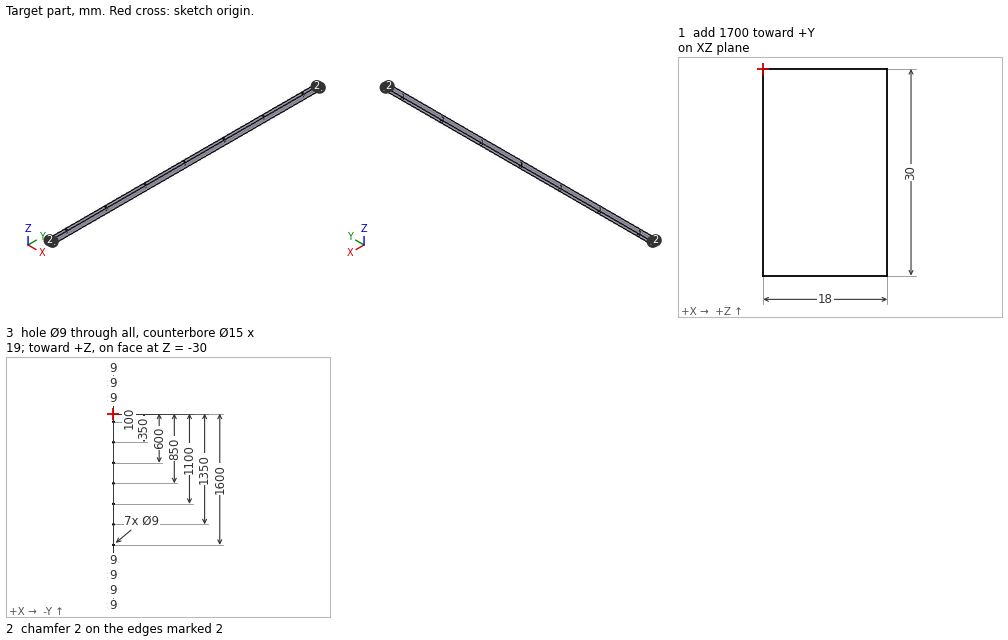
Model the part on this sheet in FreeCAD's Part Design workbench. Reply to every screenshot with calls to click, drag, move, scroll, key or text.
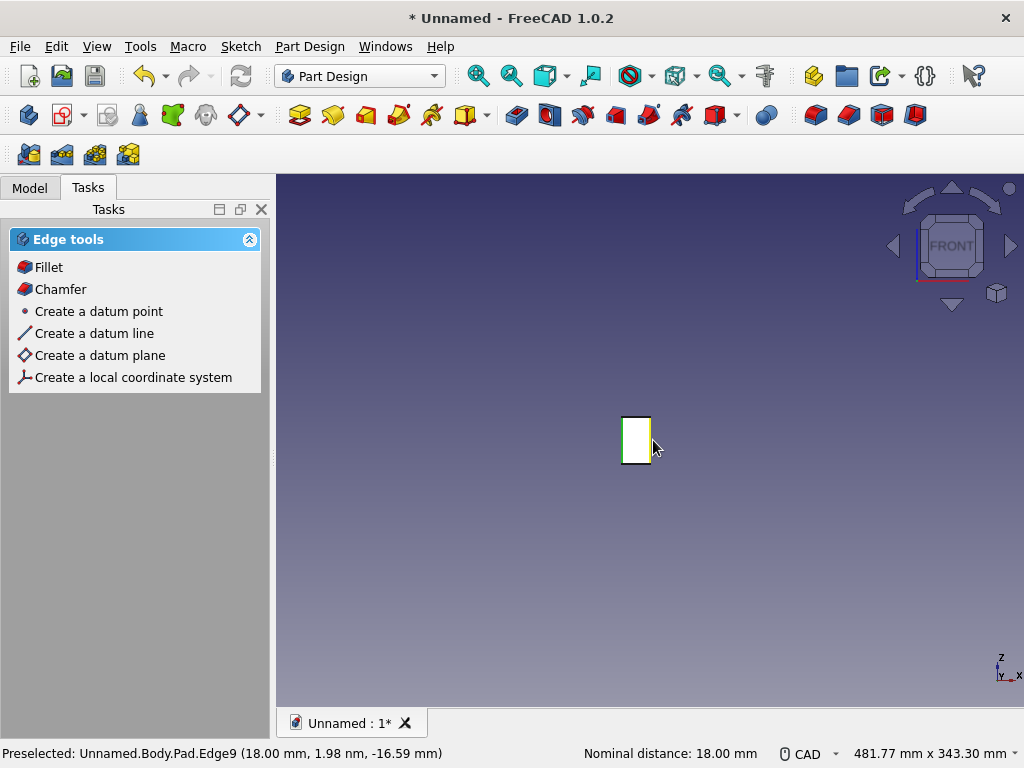
key(v)
key(f)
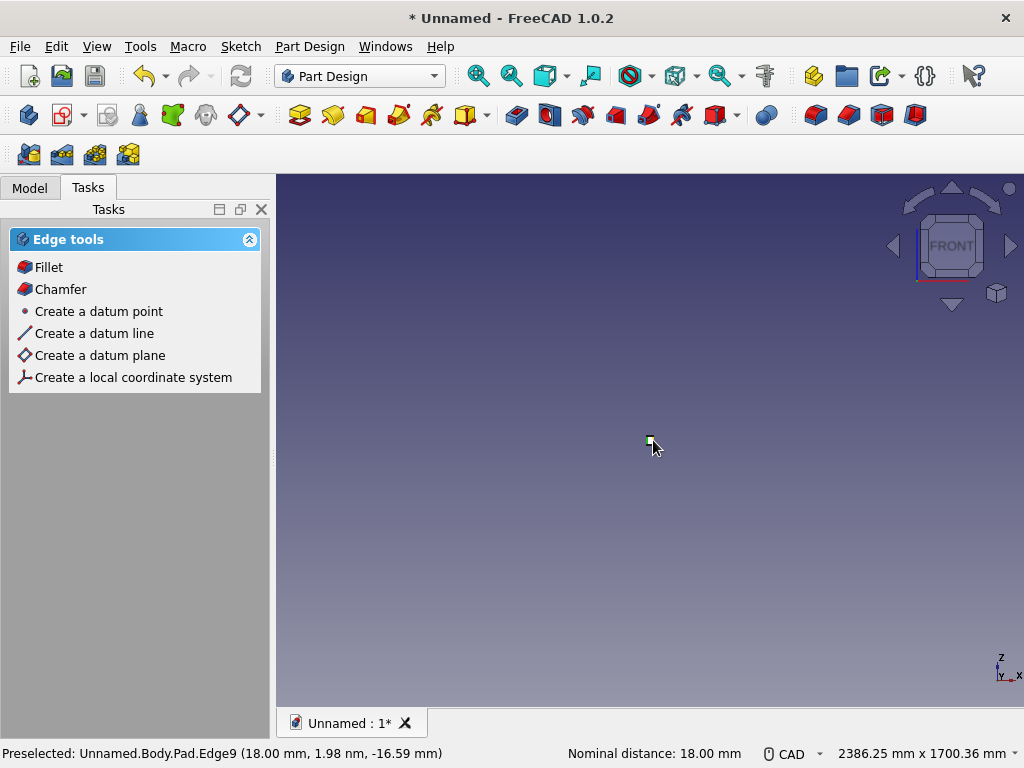
key(3)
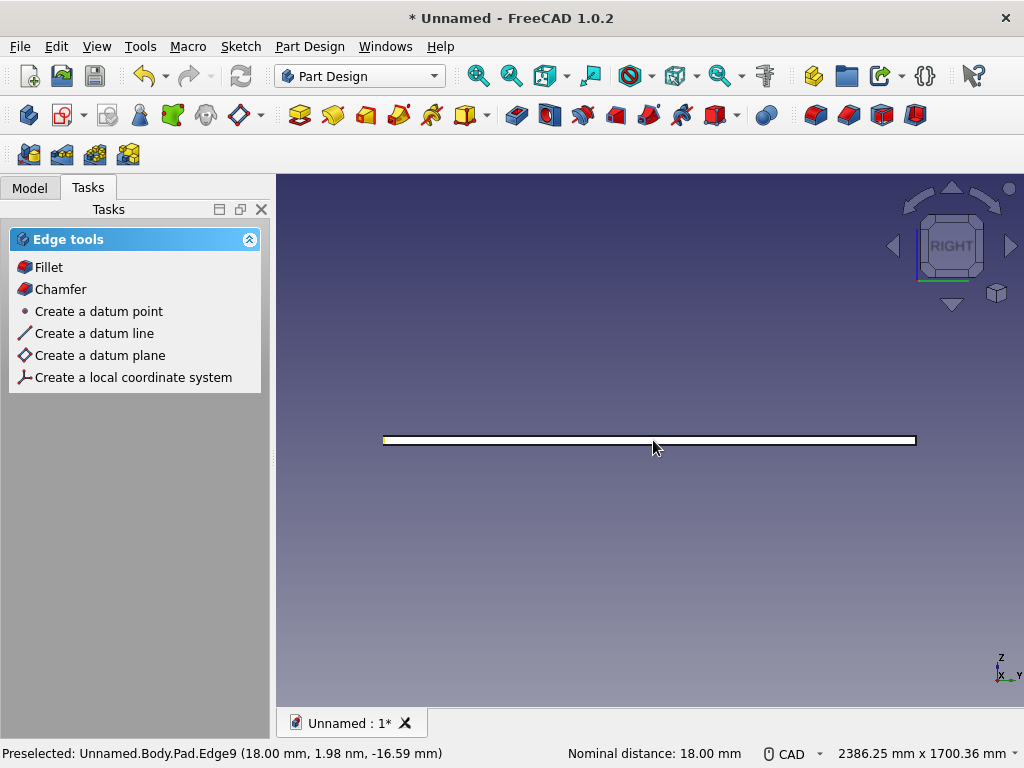
key(5)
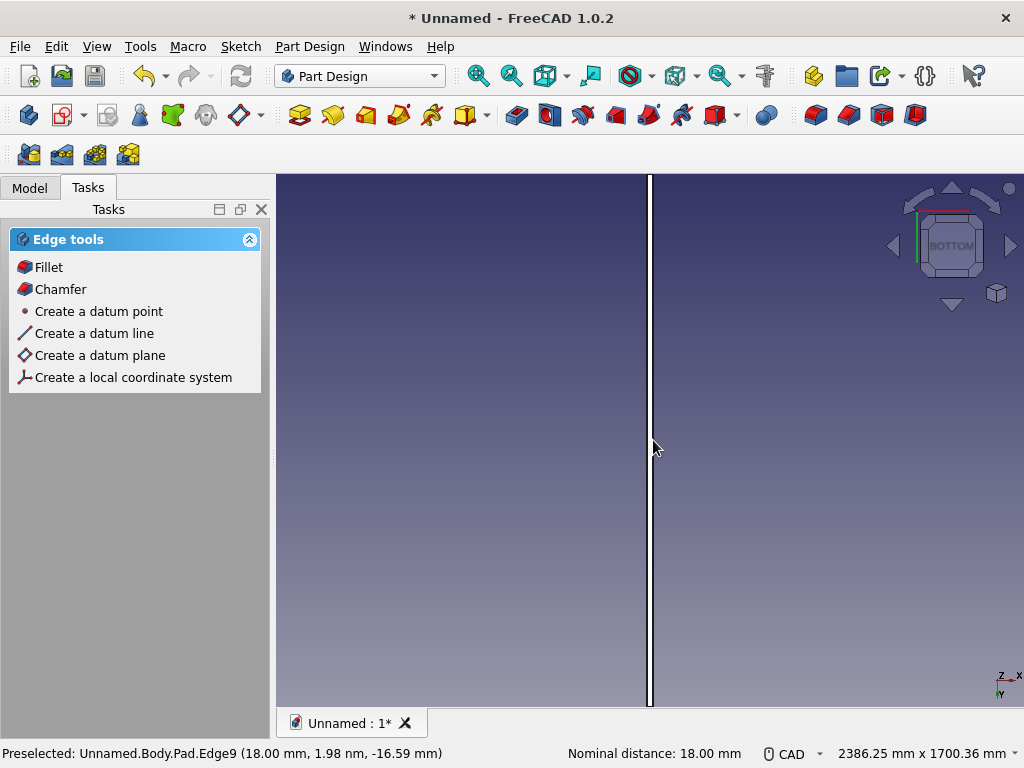
key(v)
key(f)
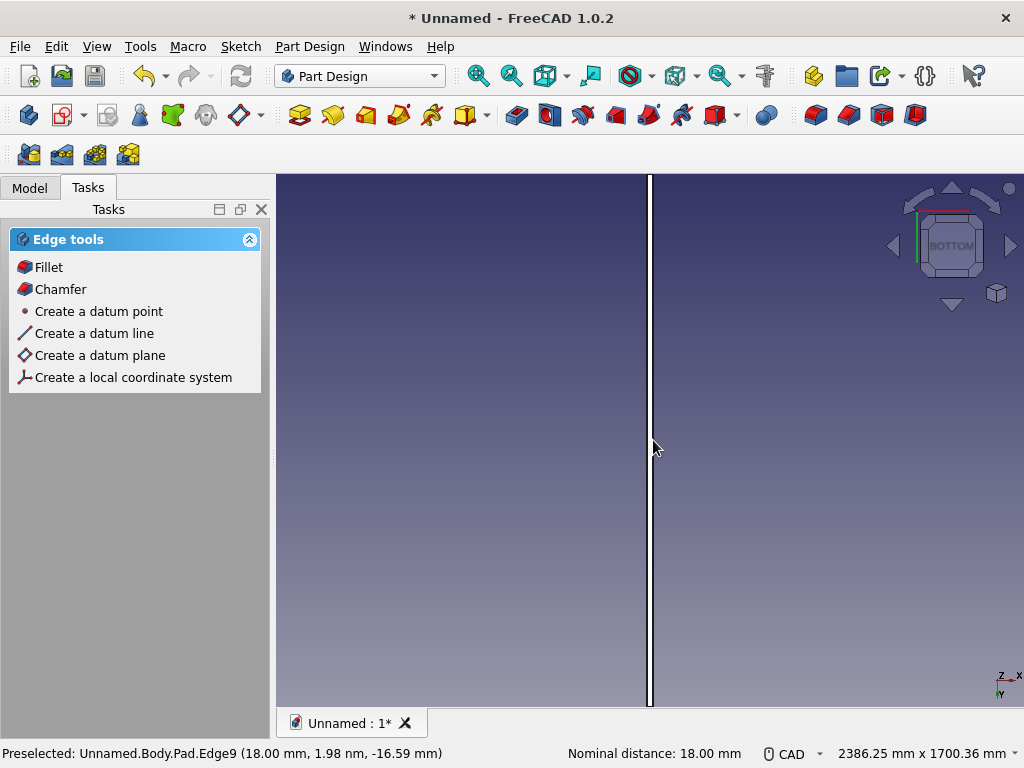
key(4)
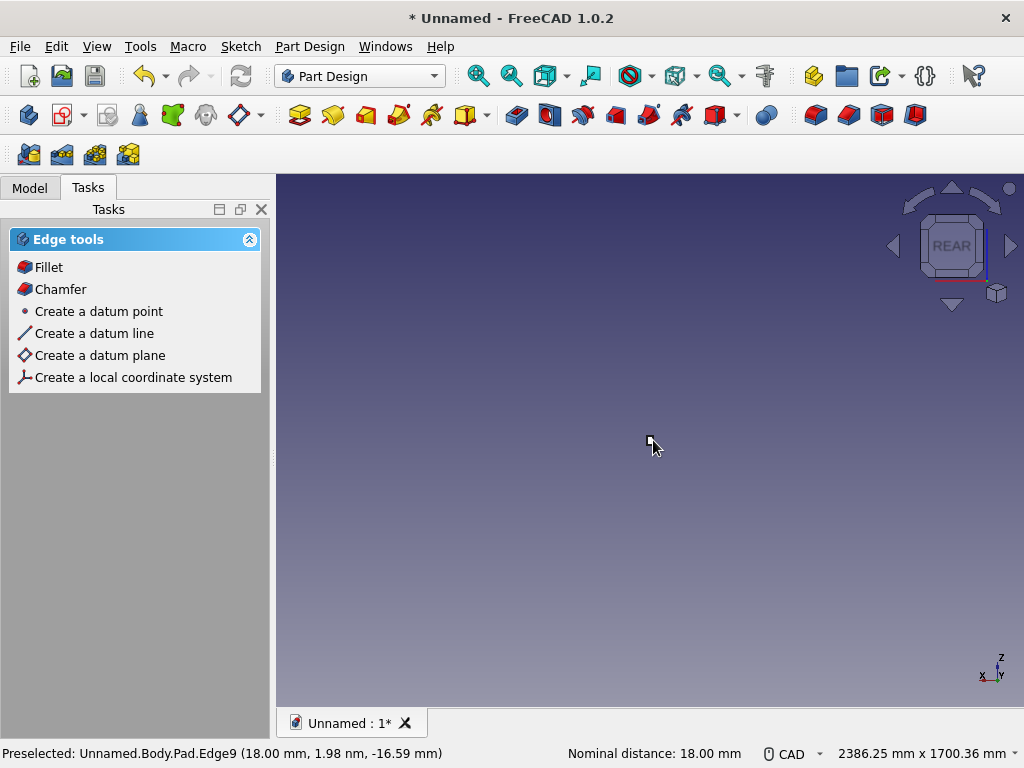
key(v)
key(f)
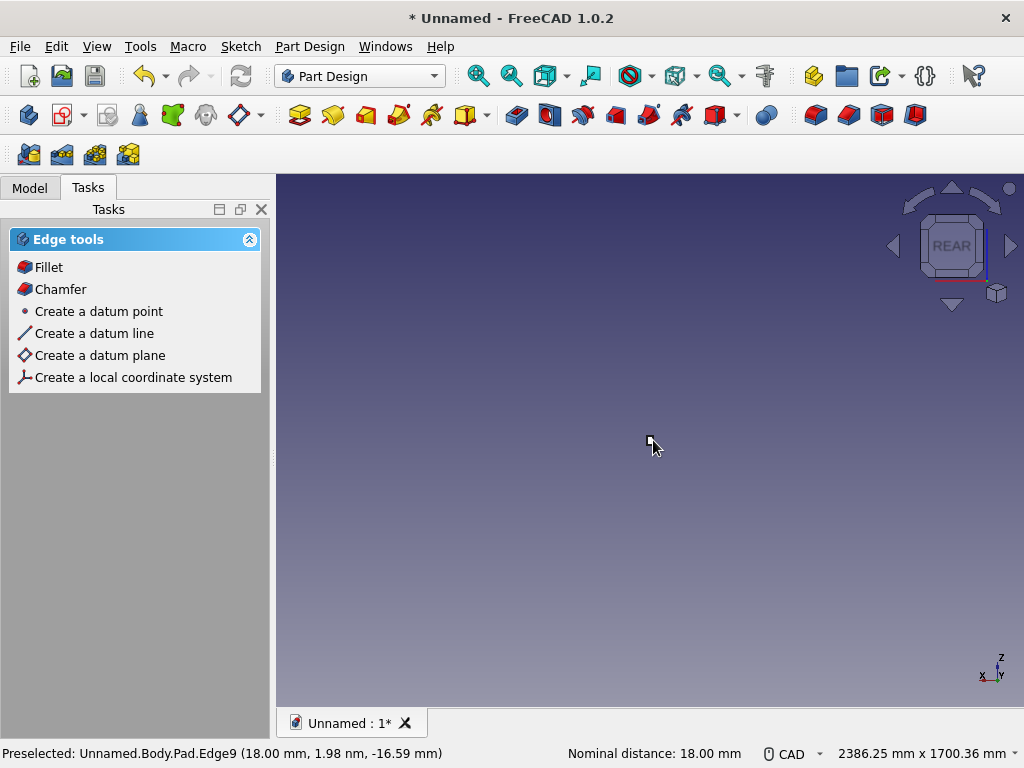
click(653, 438, ctrl)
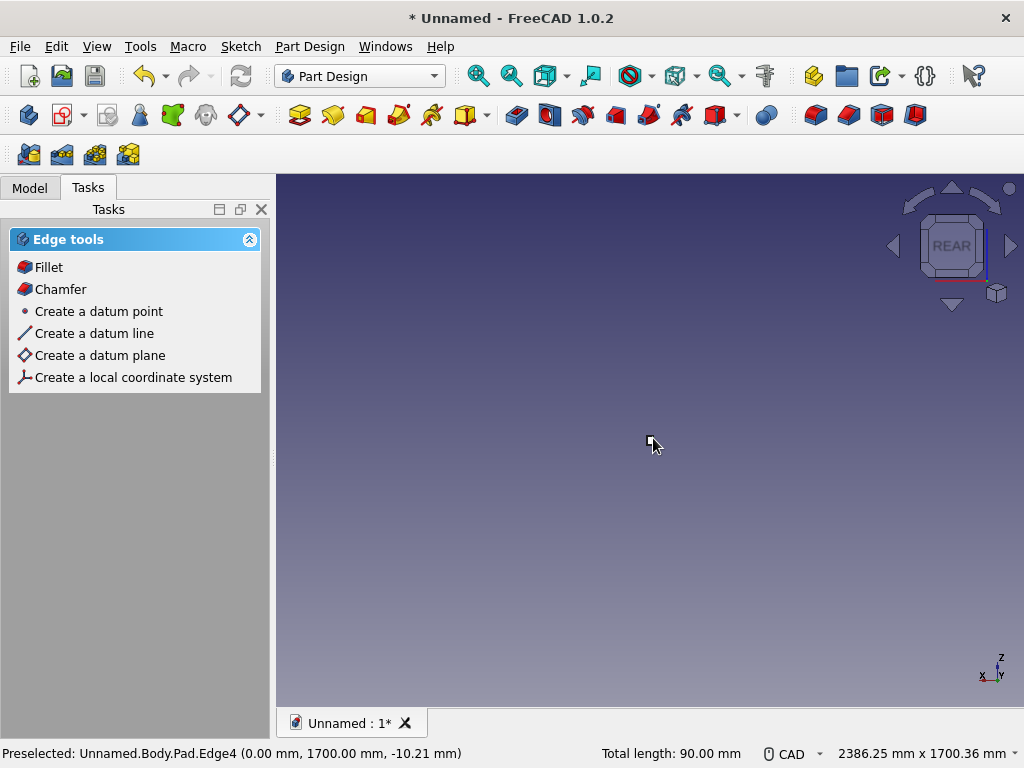
scroll(647, 440, up, 8)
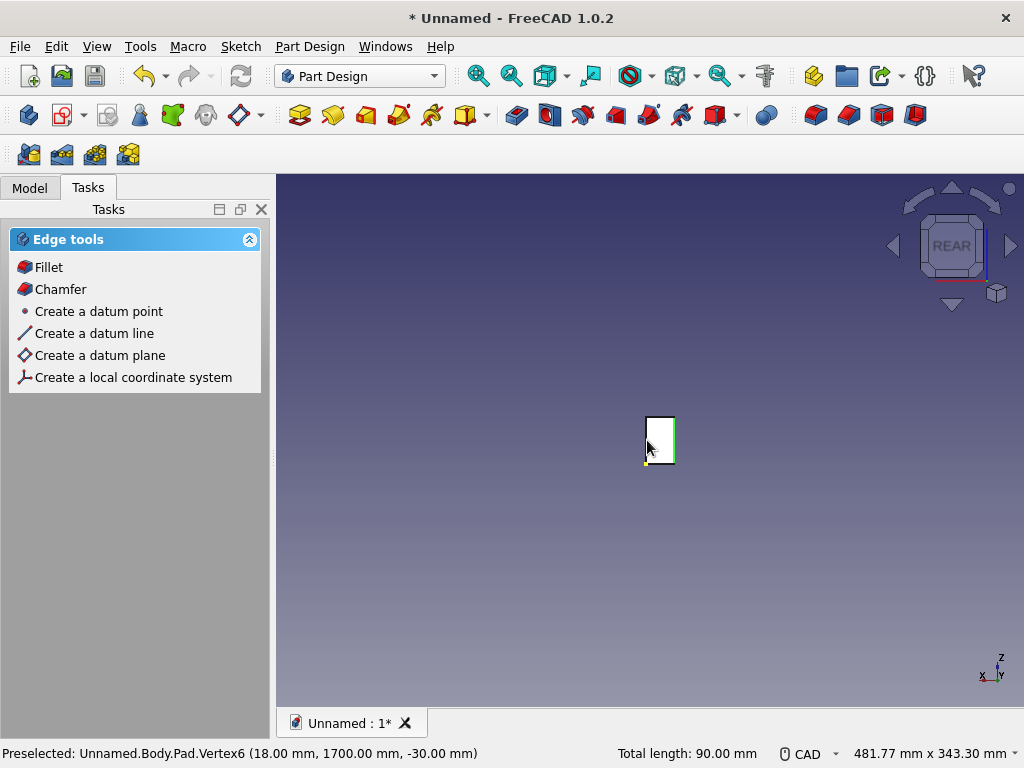
click(646, 440, ctrl)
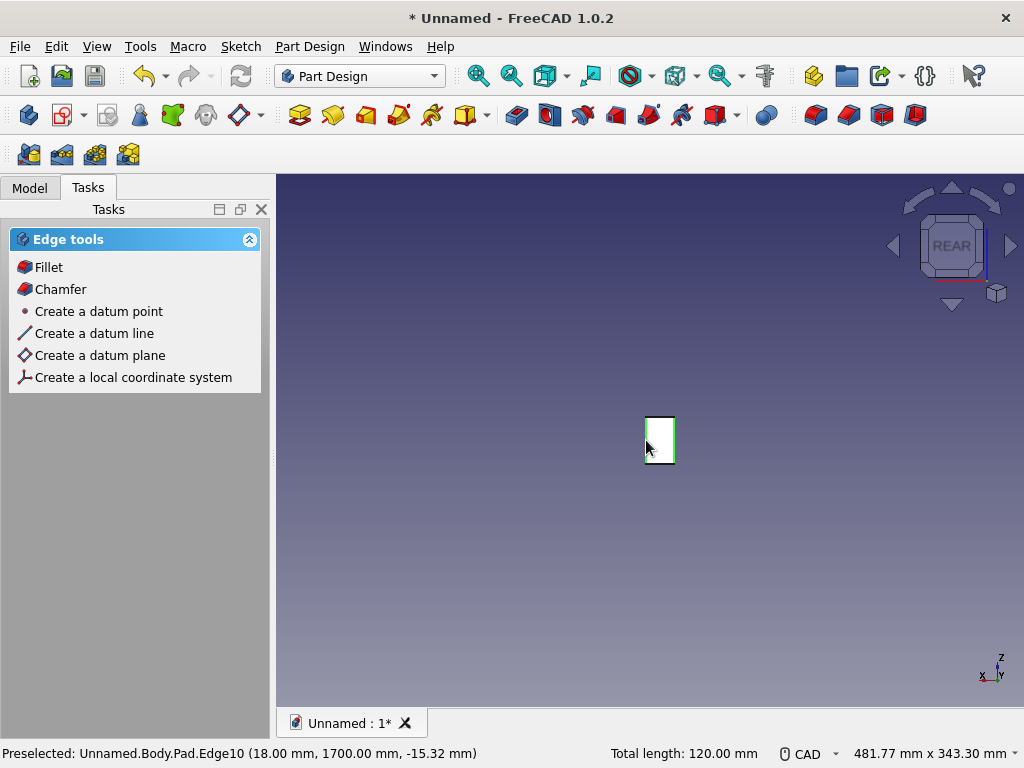
click(849, 116)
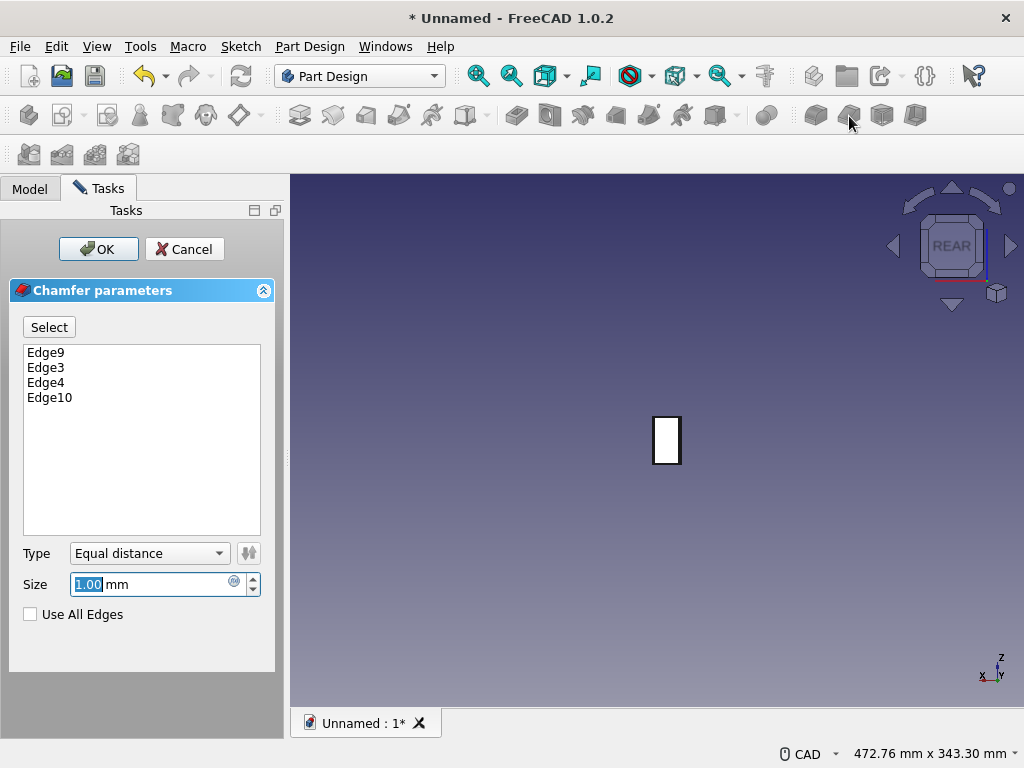
text(2)
key(Tab)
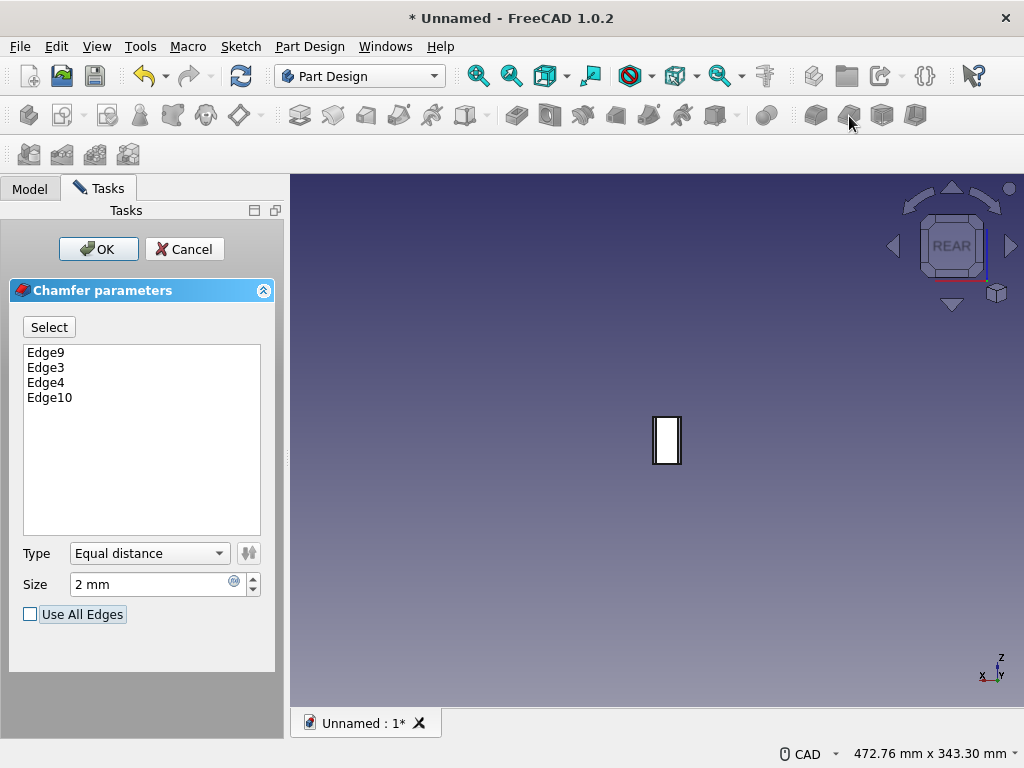
click(99, 249)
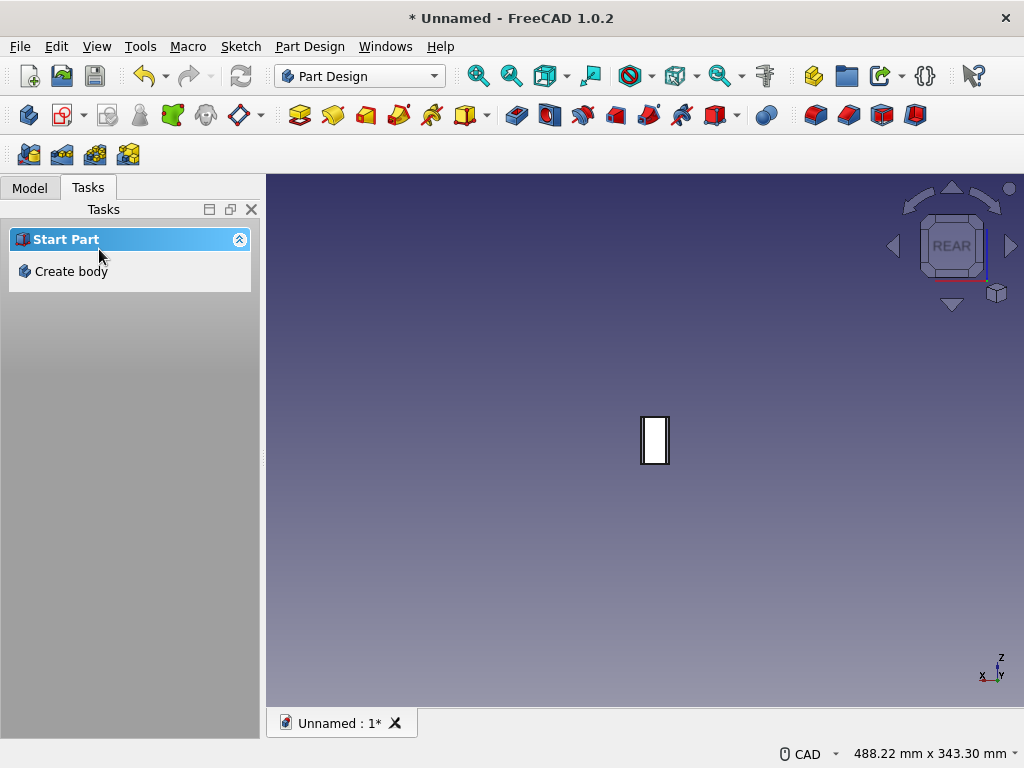
click(479, 76)